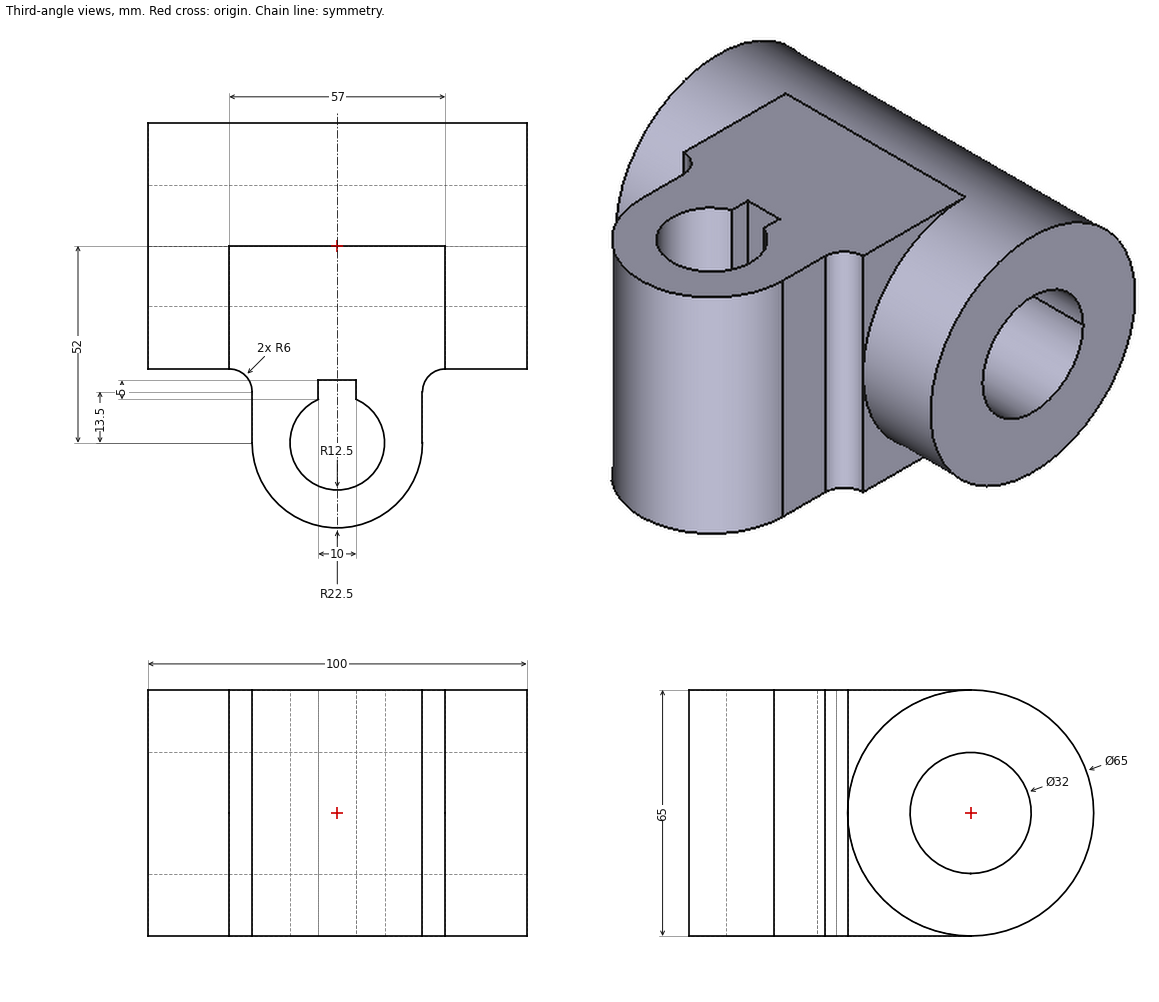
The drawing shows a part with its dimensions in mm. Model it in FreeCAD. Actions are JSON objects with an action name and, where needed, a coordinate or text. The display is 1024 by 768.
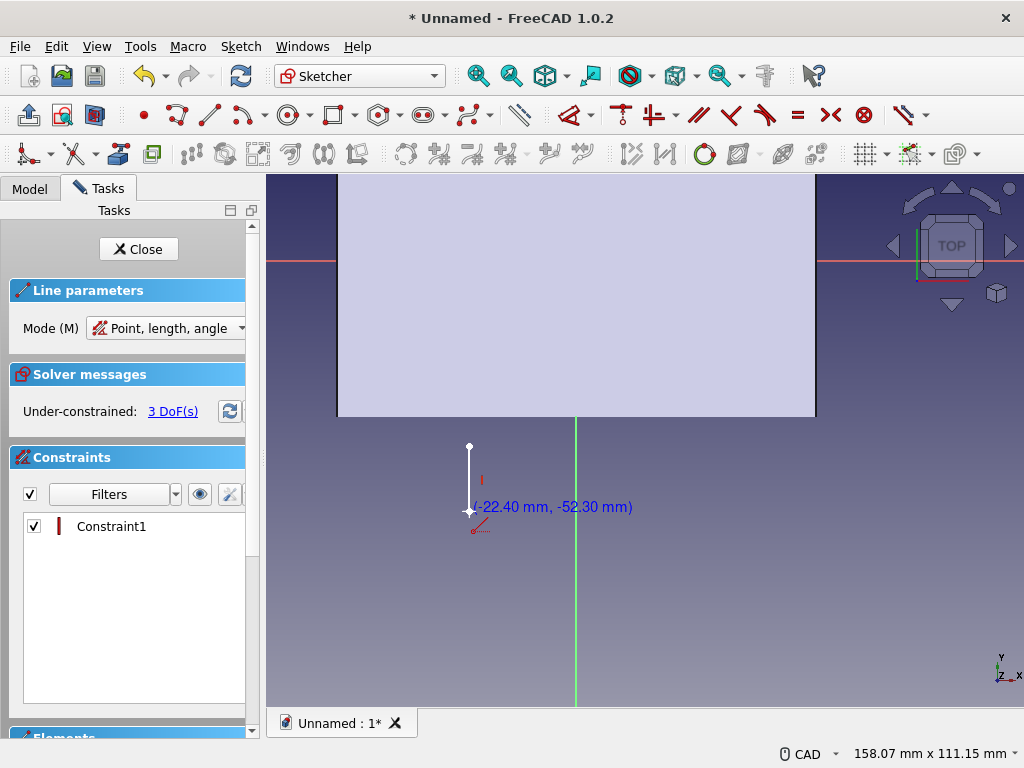
{"action": "left_click", "coordinate": [684, 511]}
{"action": "left_click", "coordinate": [684, 446]}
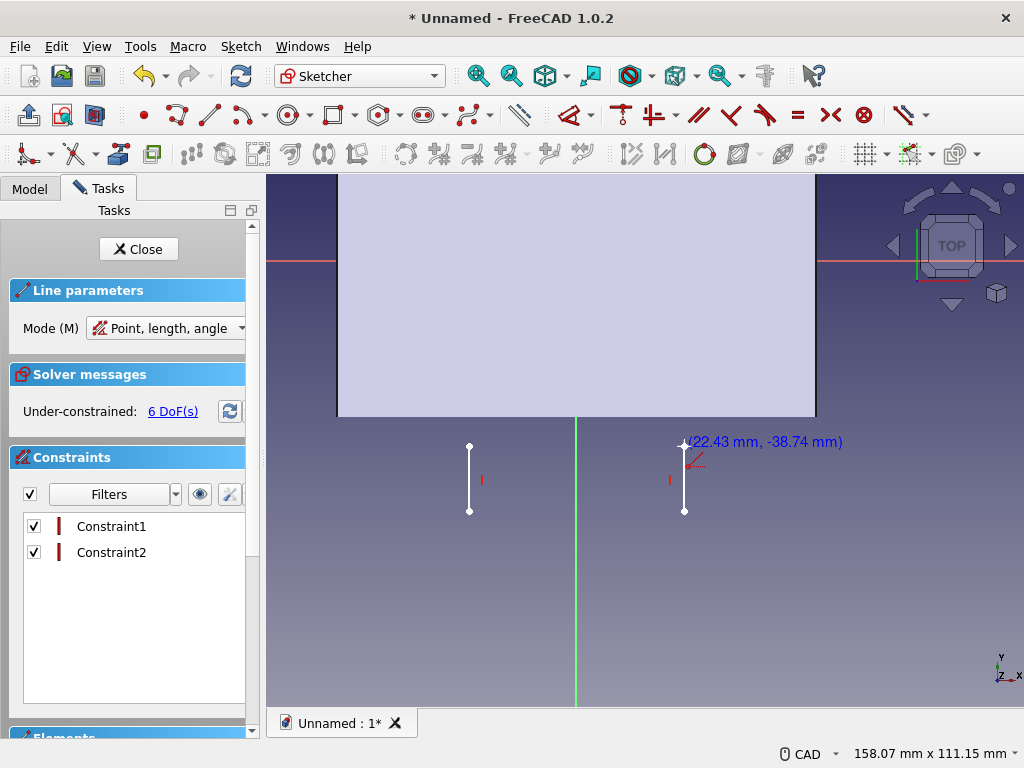
{"action": "left_click", "coordinate": [713, 417]}
{"action": "left_click", "coordinate": [440, 417]}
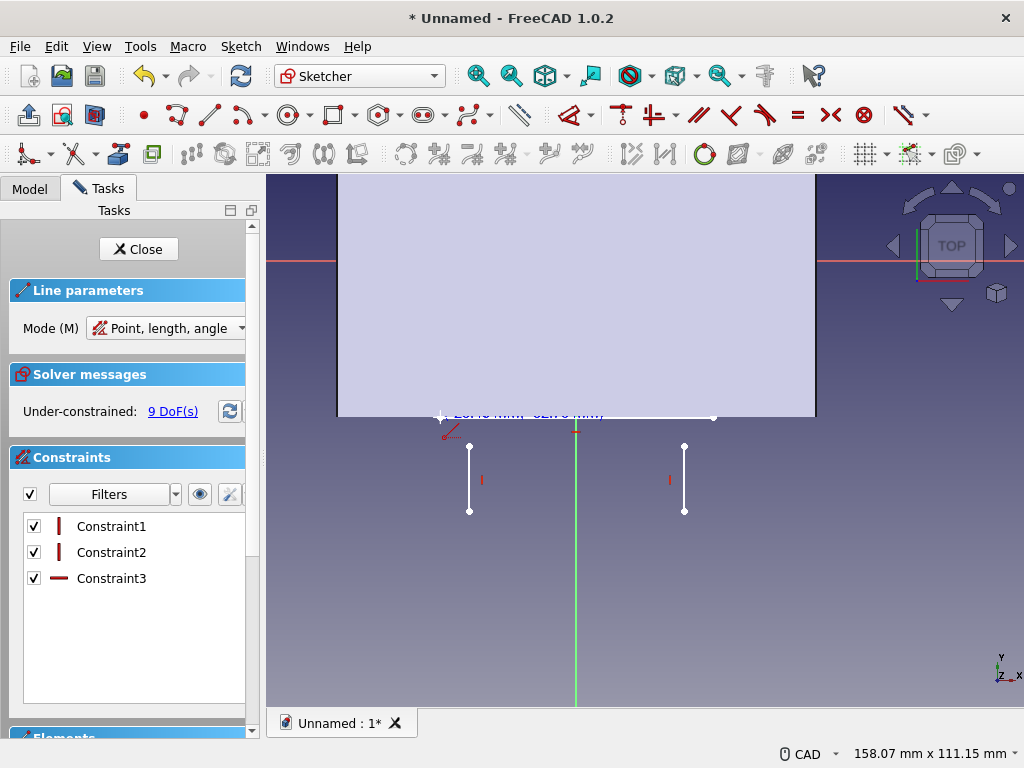
{"action": "left_click", "coordinate": [264, 116]}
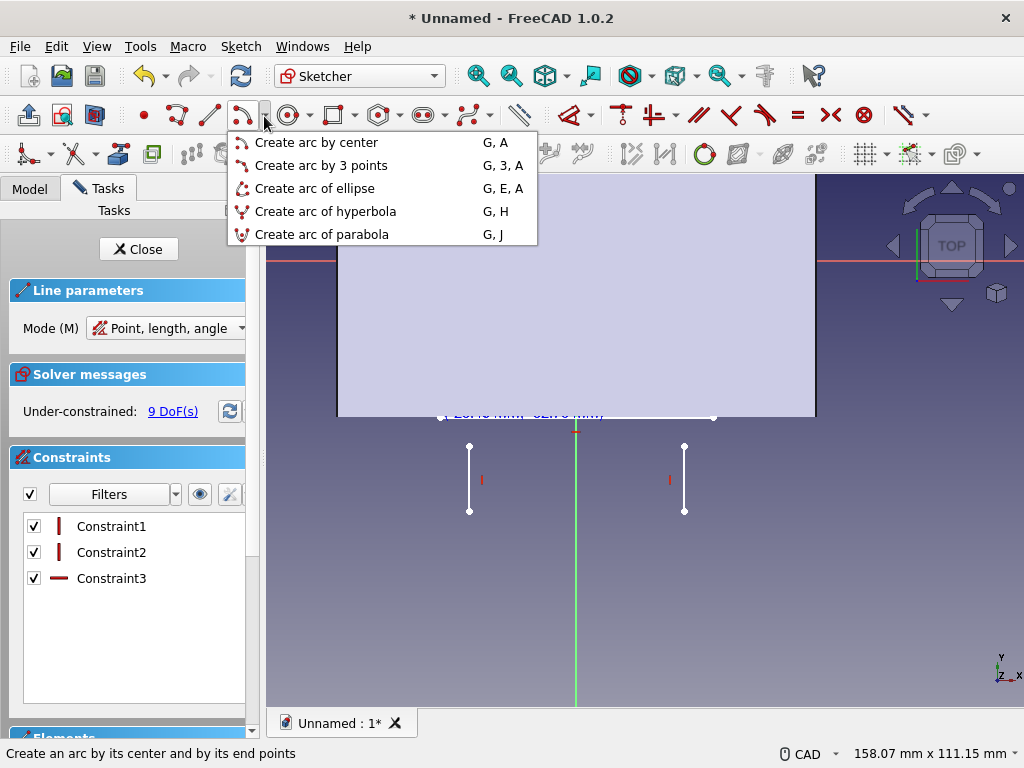
{"action": "left_click", "coordinate": [382, 166]}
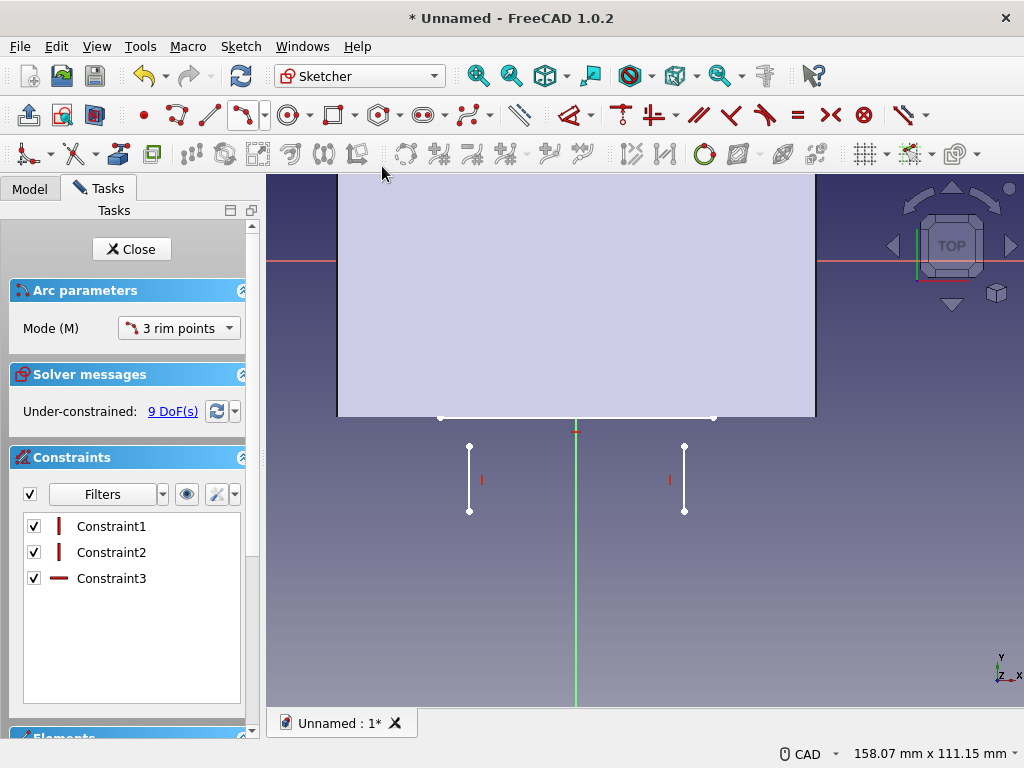
{"action": "left_click", "coordinate": [469, 512]}
{"action": "left_click", "coordinate": [684, 512]}
{"action": "left_click", "coordinate": [543, 613]}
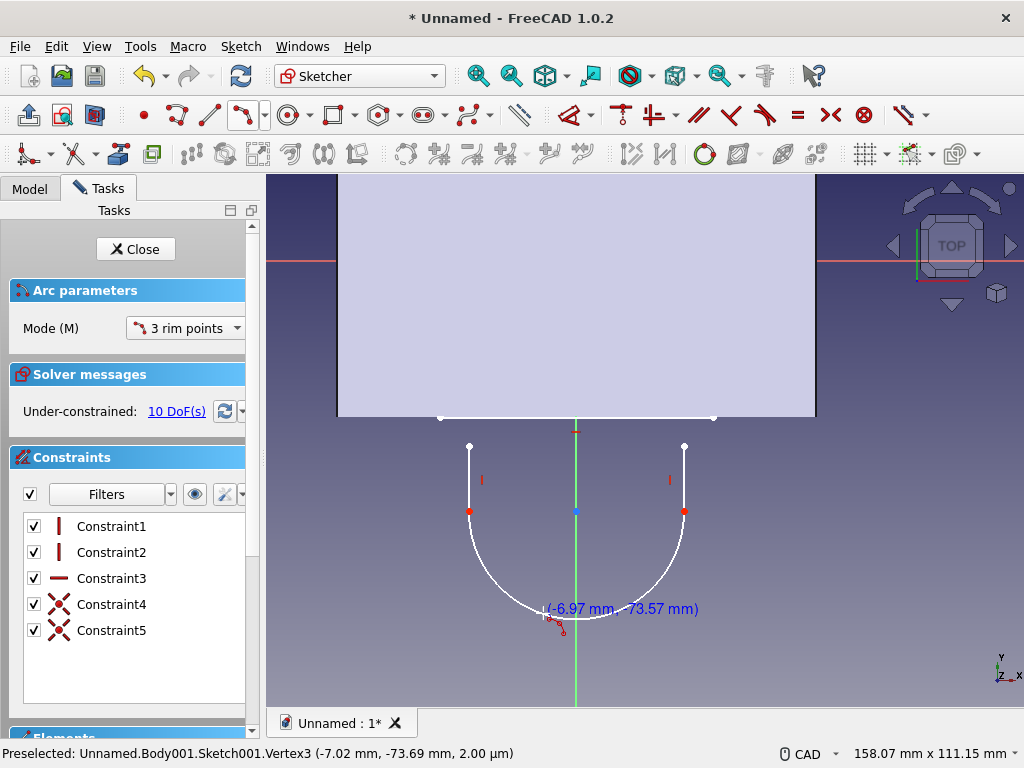
{"action": "left_click", "coordinate": [684, 447]}
{"action": "left_click", "coordinate": [713, 418]}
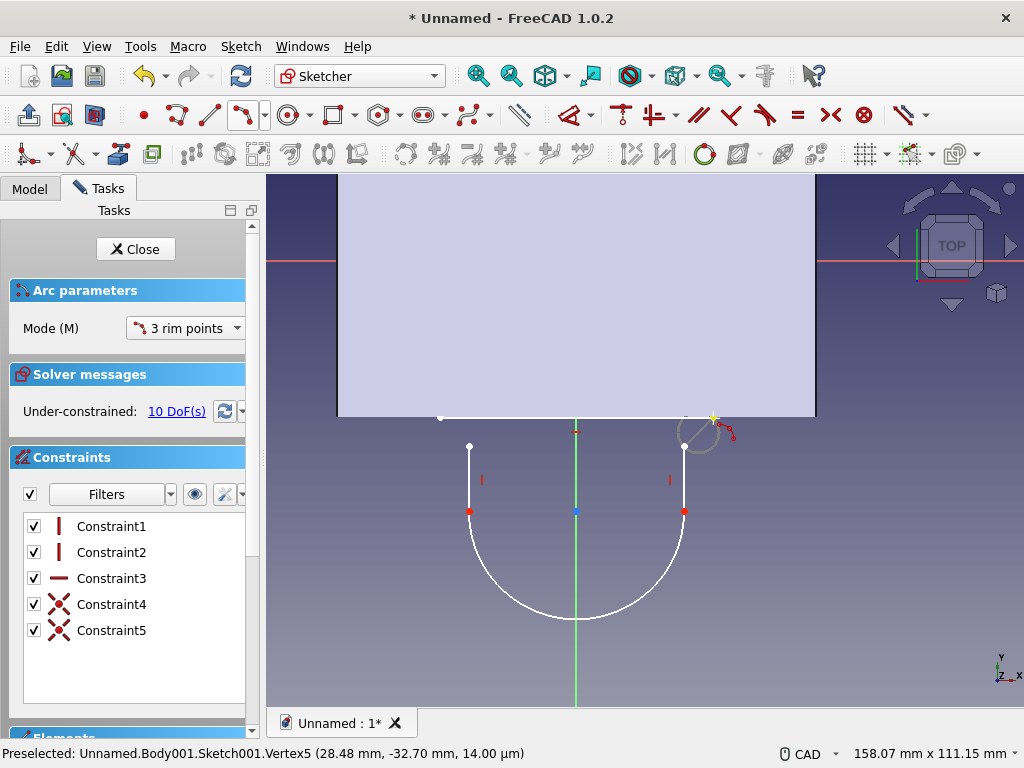
{"action": "scroll", "coordinate": [693, 425], "scroll_direction": "up", "scroll_amount": 4}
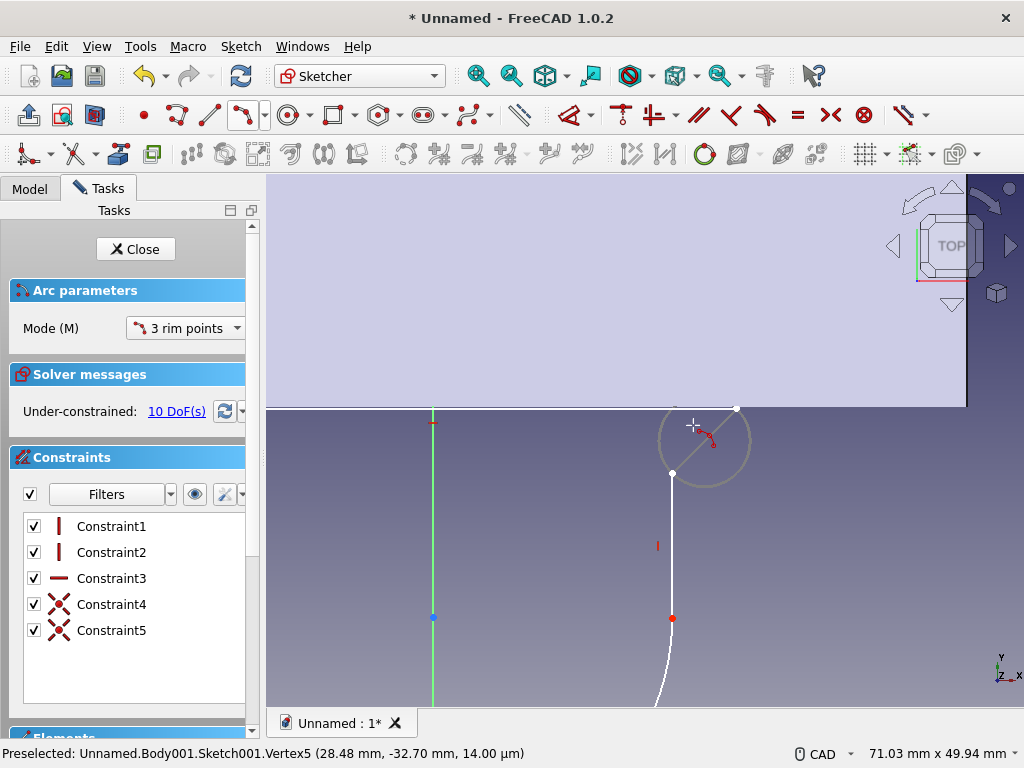
{"action": "left_click", "coordinate": [692, 425]}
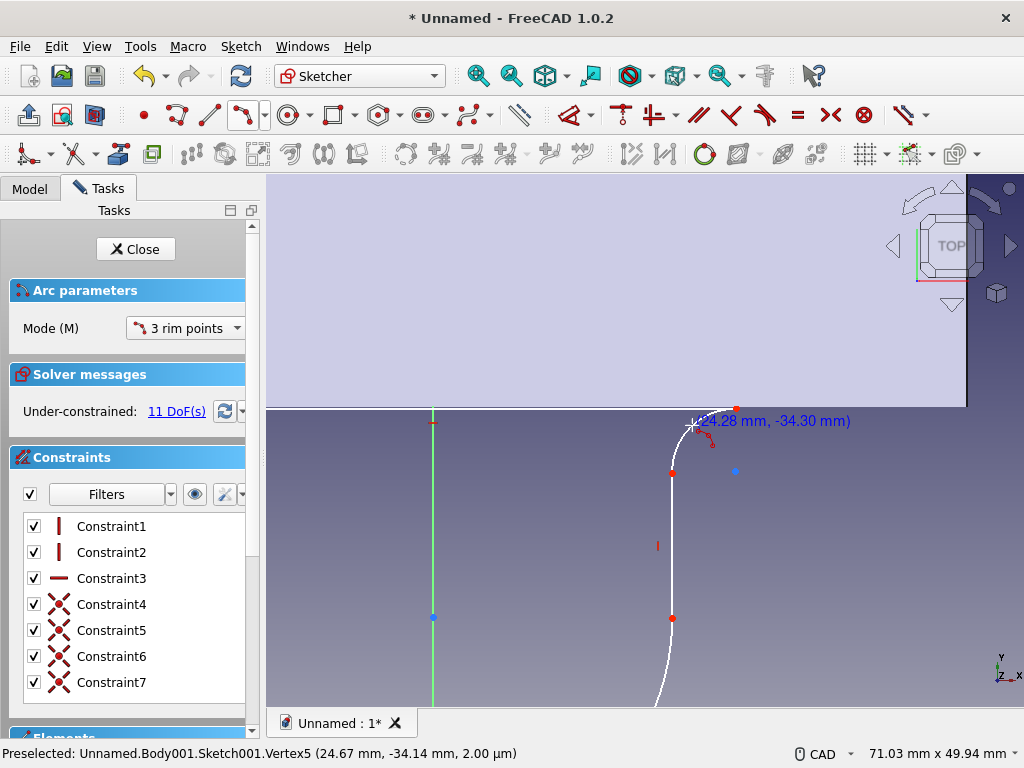
{"action": "scroll", "coordinate": [694, 427], "scroll_direction": "down", "scroll_amount": 4}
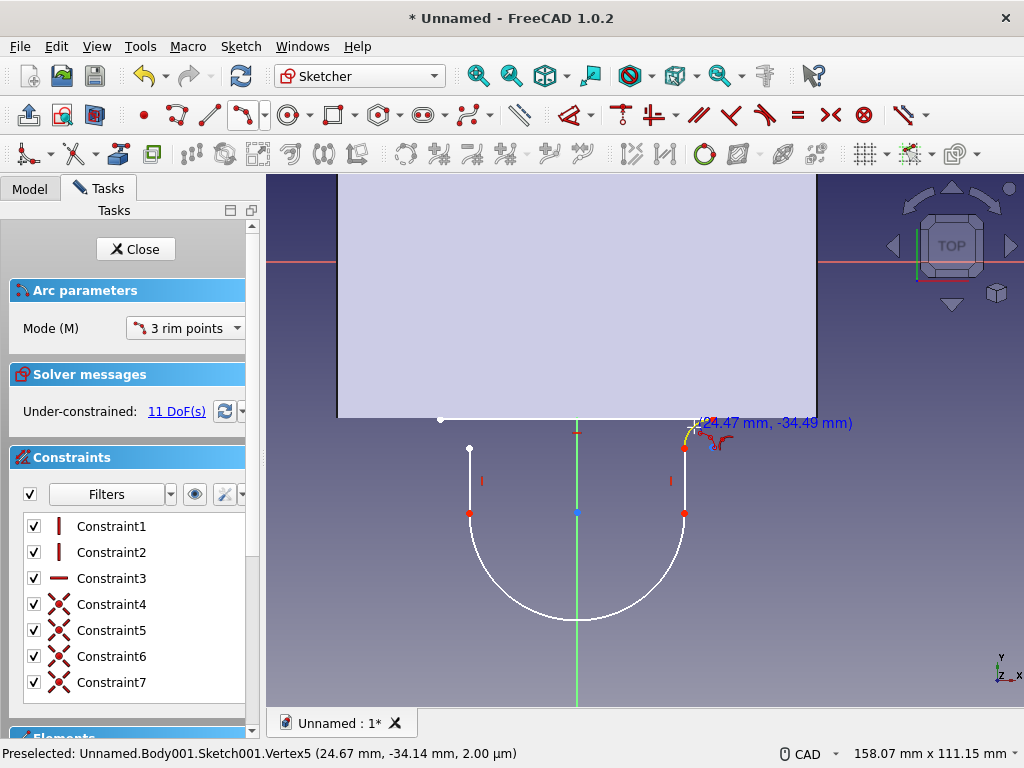
{"action": "left_click", "coordinate": [441, 419]}
{"action": "left_click", "coordinate": [470, 448]}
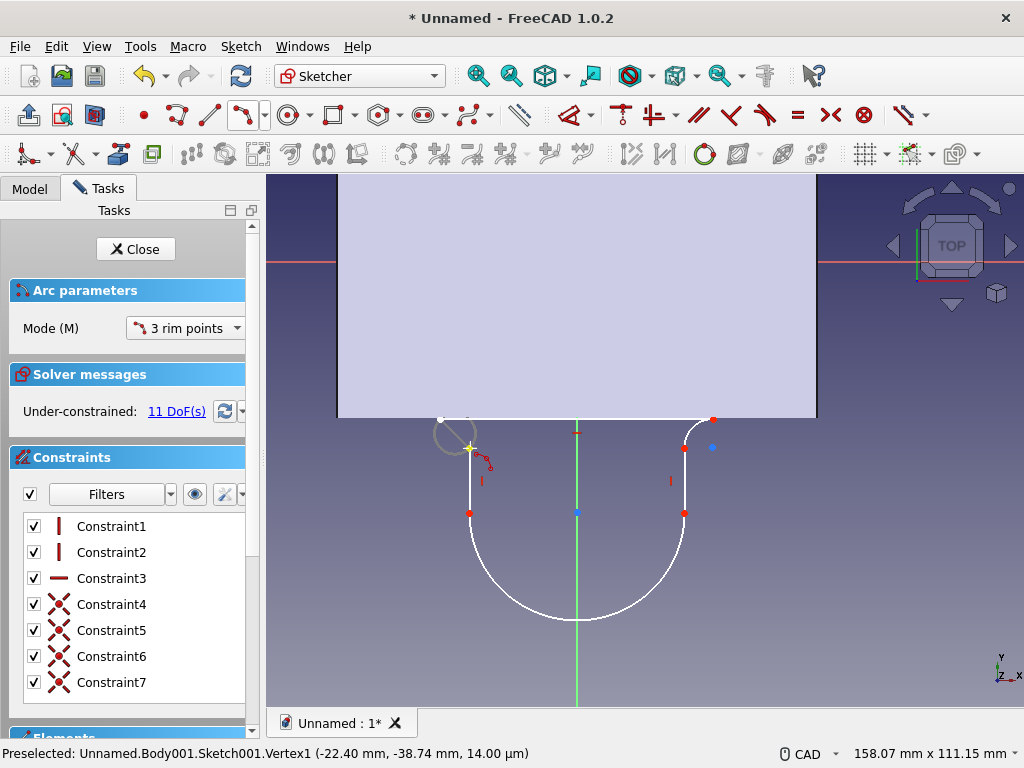
{"action": "scroll", "coordinate": [461, 427], "scroll_direction": "up", "scroll_amount": 4}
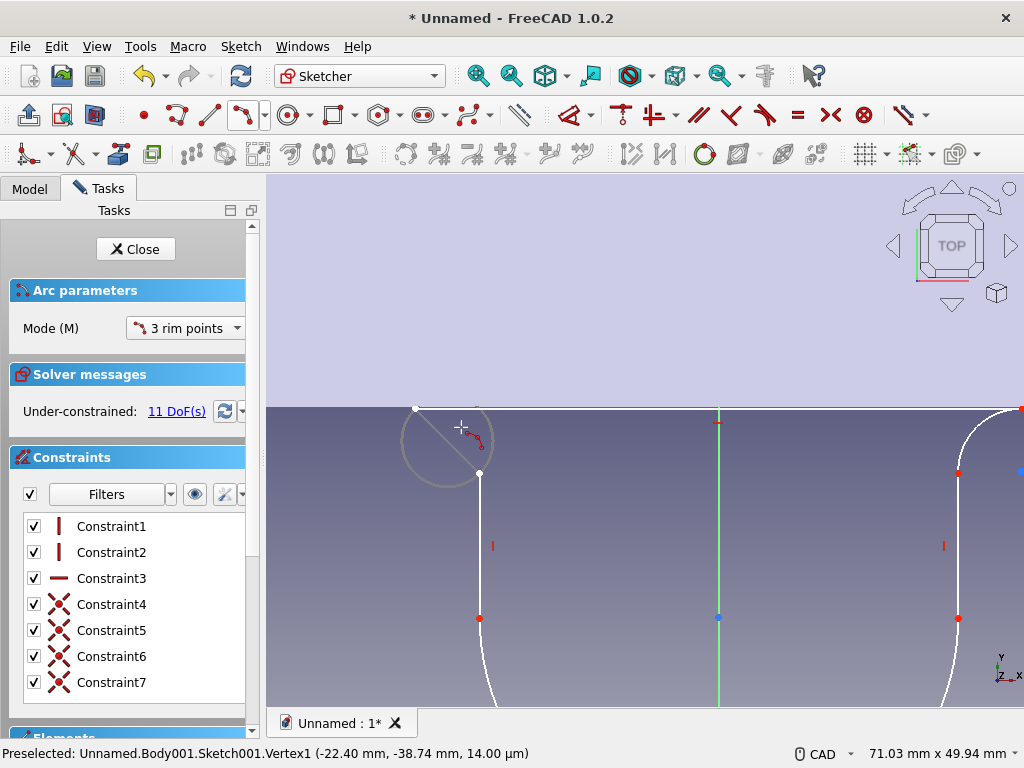
{"action": "left_click", "coordinate": [460, 425]}